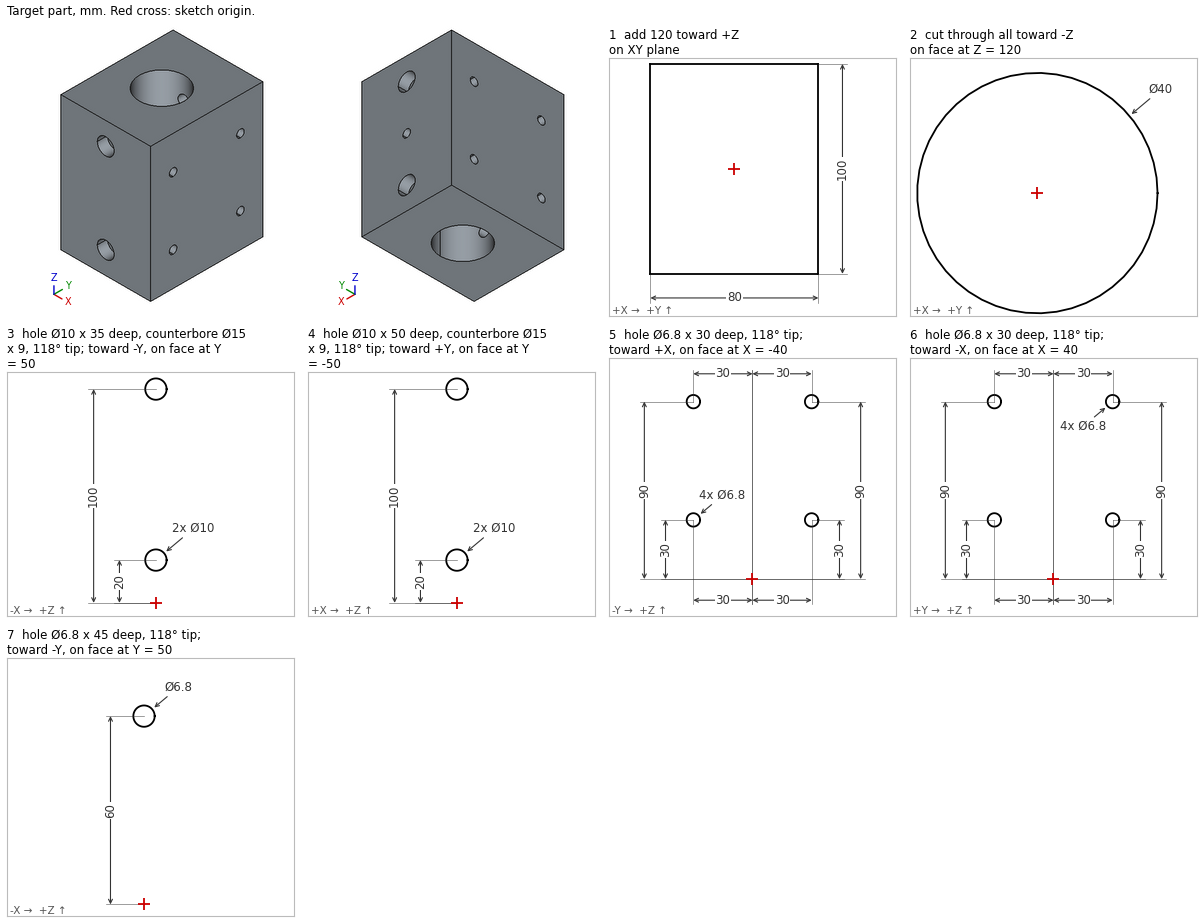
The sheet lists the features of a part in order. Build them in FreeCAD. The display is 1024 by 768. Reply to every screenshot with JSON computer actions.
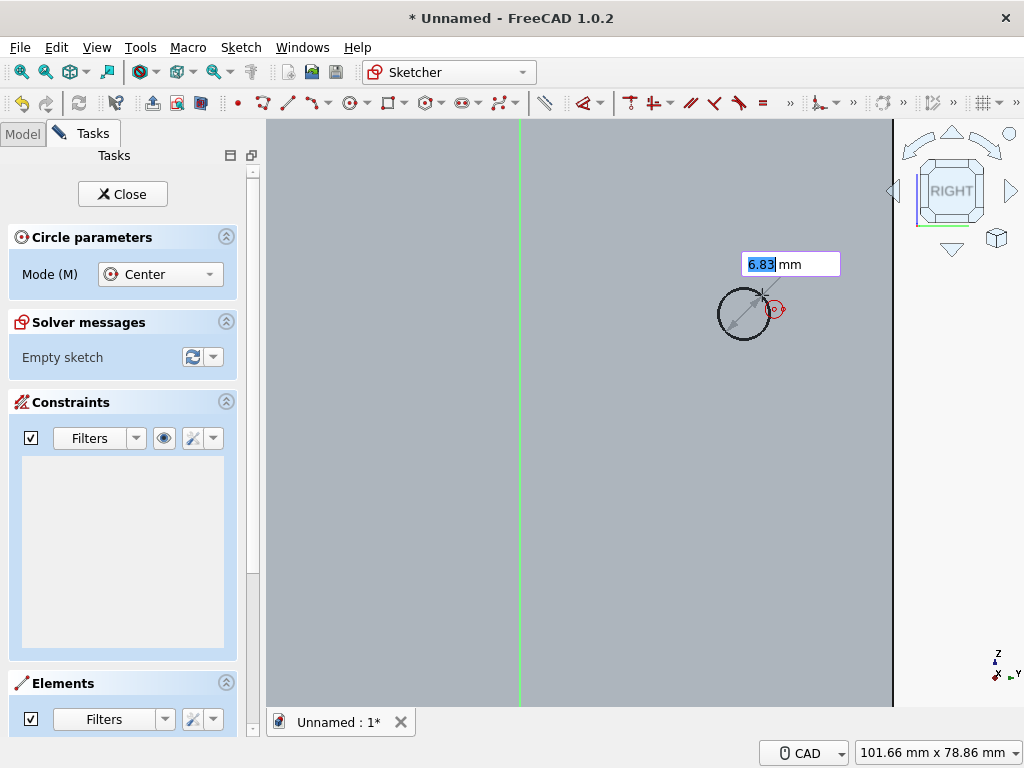
{"action": "type", "text": "6.8"}
{"action": "key", "text": "Return"}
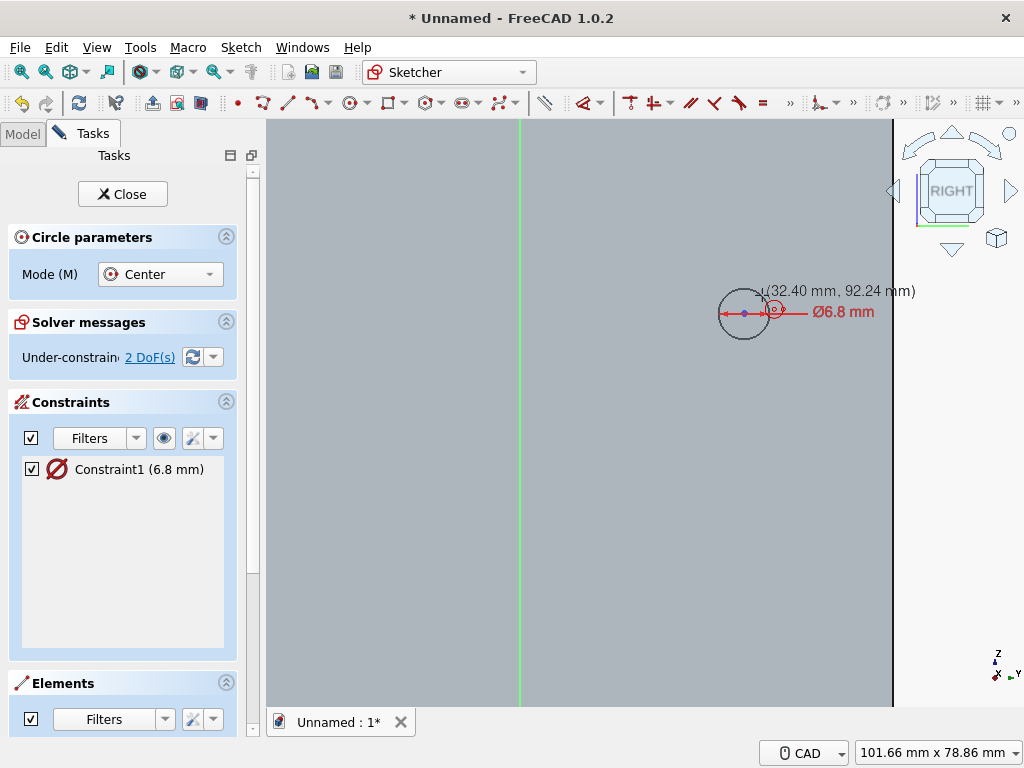
{"action": "scroll", "coordinate": [645, 147], "scroll_direction": "down", "scroll_amount": 3}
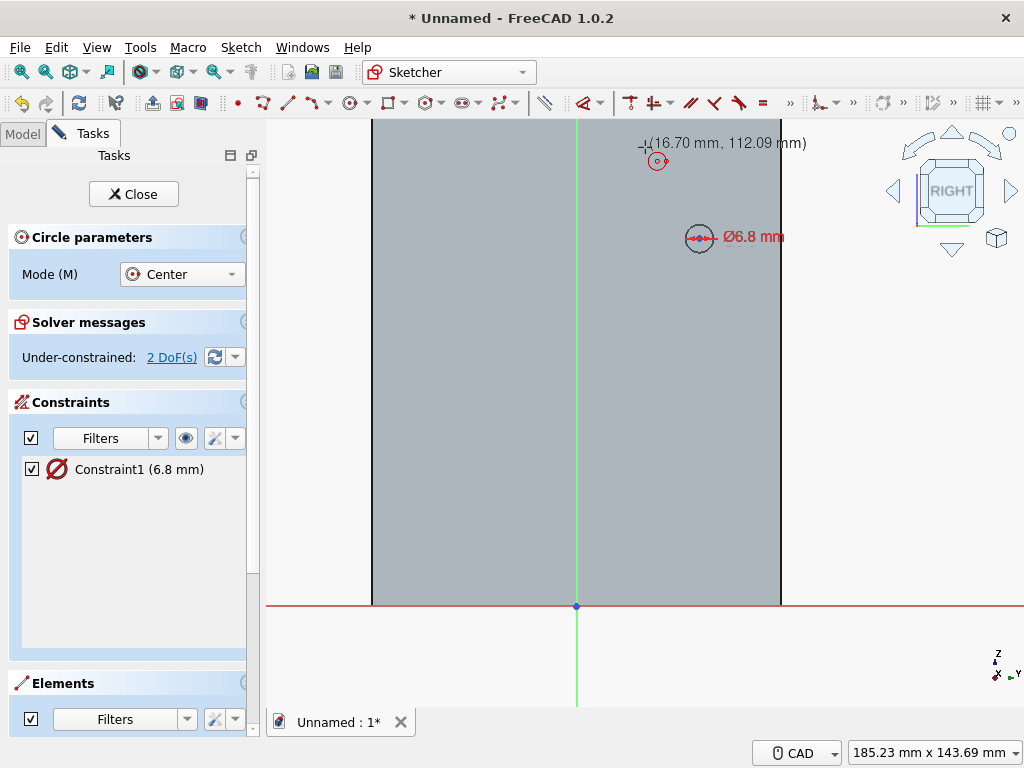
{"action": "scroll", "coordinate": [700, 483], "scroll_direction": "up", "scroll_amount": 3}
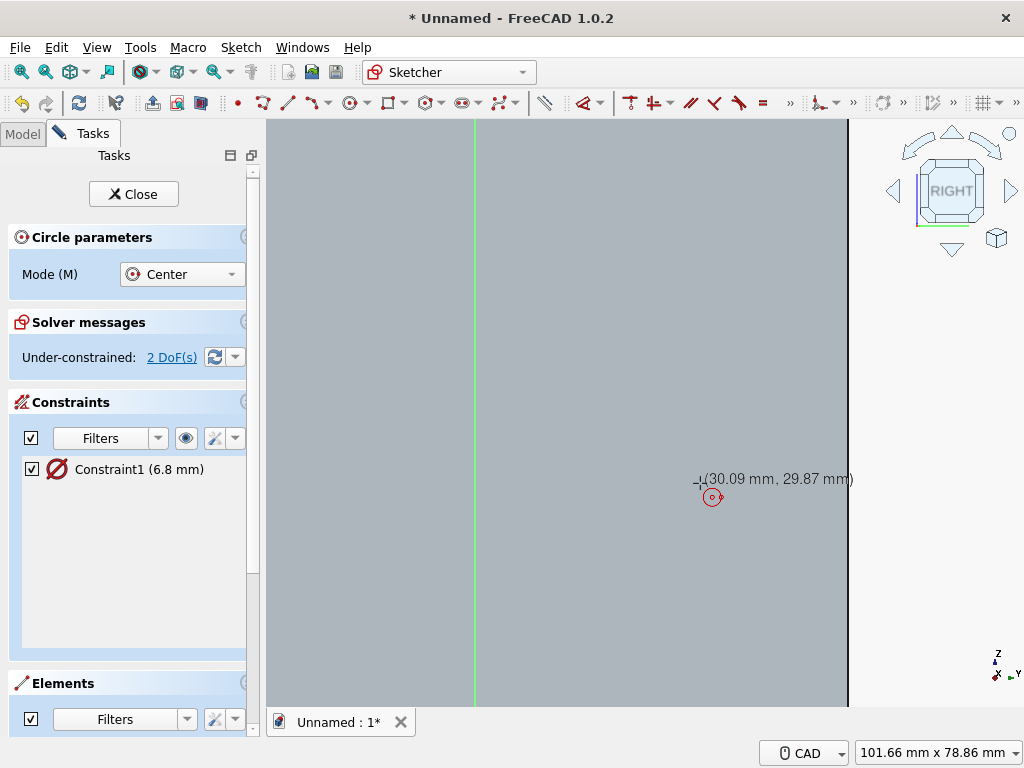
{"action": "left_click", "coordinate": [699, 483]}
{"action": "mouse_move", "coordinate": [717, 465]}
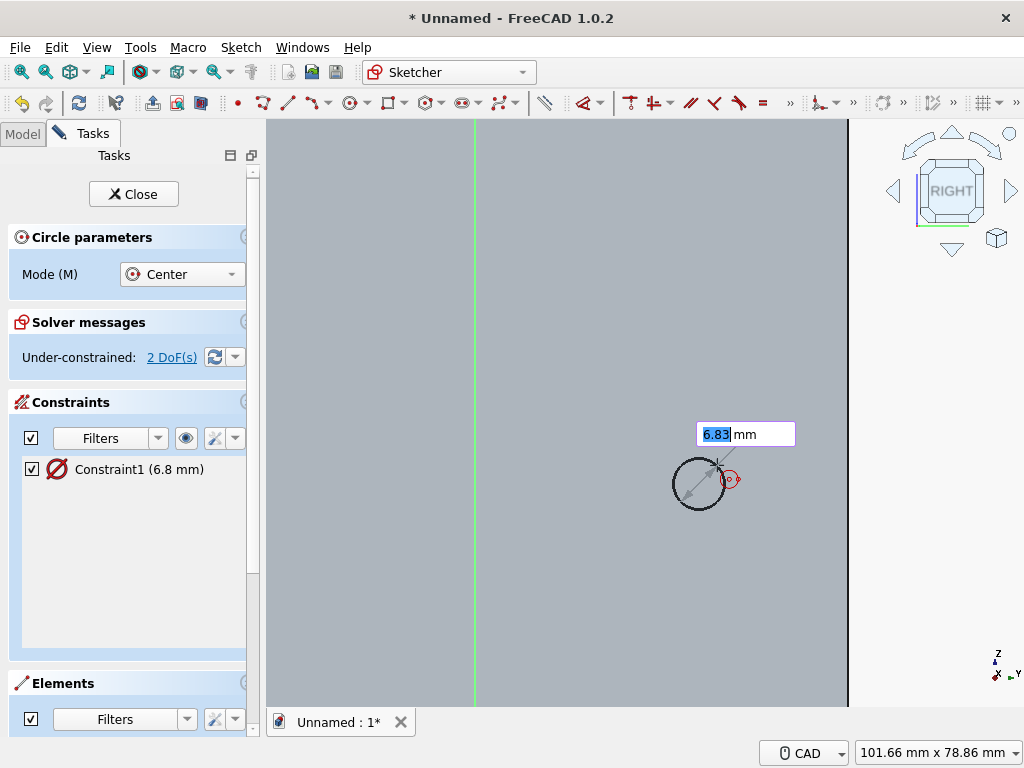
{"action": "type", "text": "6.8"}
{"action": "key", "text": "Return"}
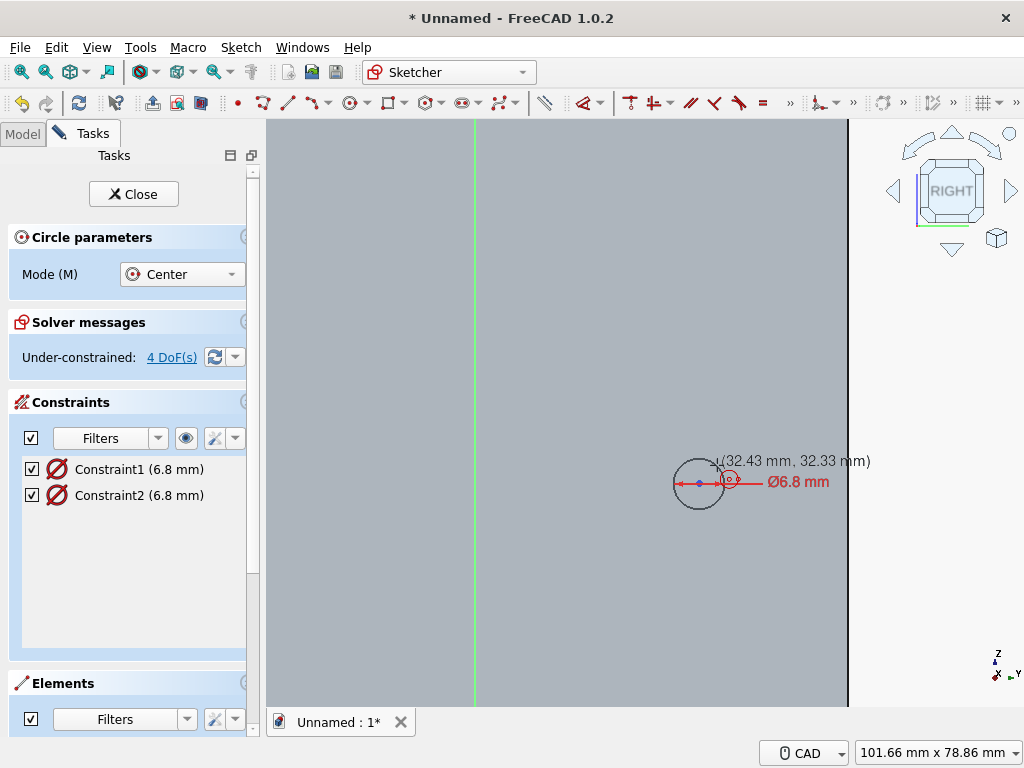
{"action": "scroll", "coordinate": [700, 479], "scroll_direction": "down", "scroll_amount": 3}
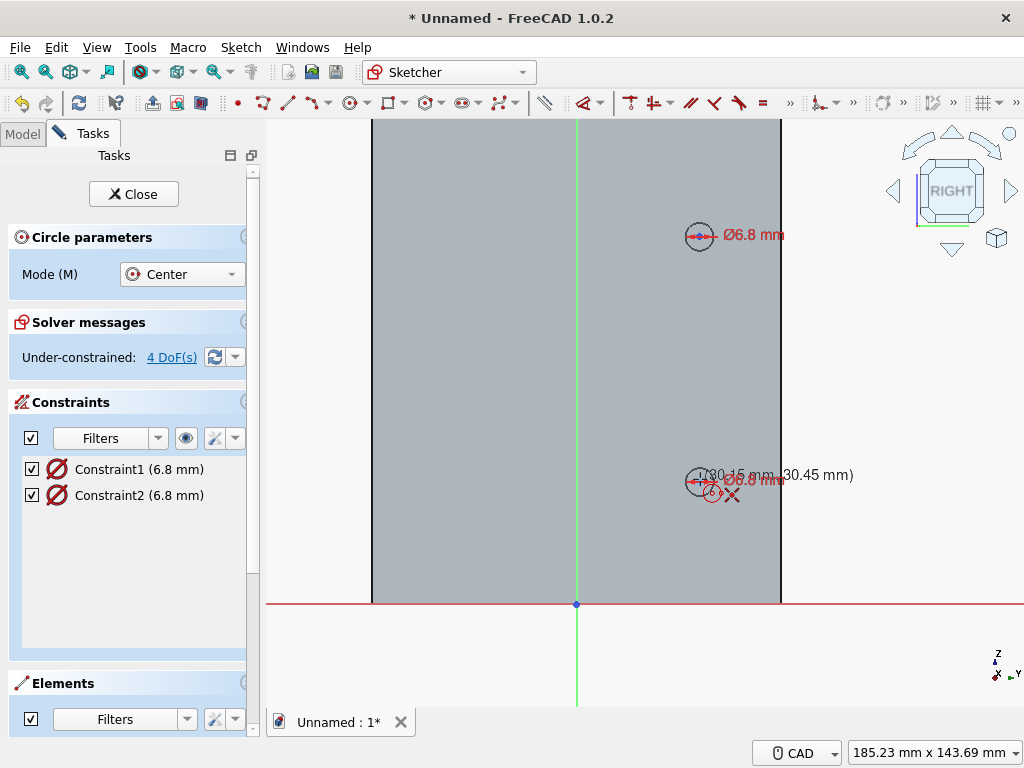
{"action": "scroll", "coordinate": [454, 482], "scroll_direction": "up", "scroll_amount": 3}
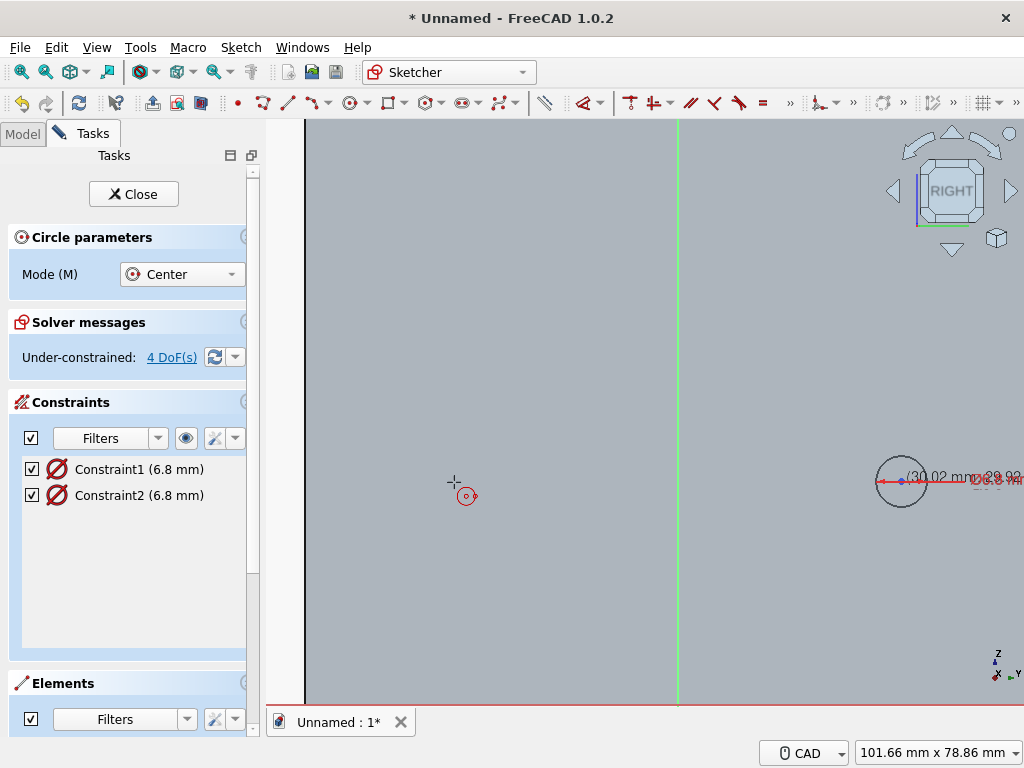
{"action": "left_click", "coordinate": [454, 481]}
{"action": "mouse_move", "coordinate": [472, 463]}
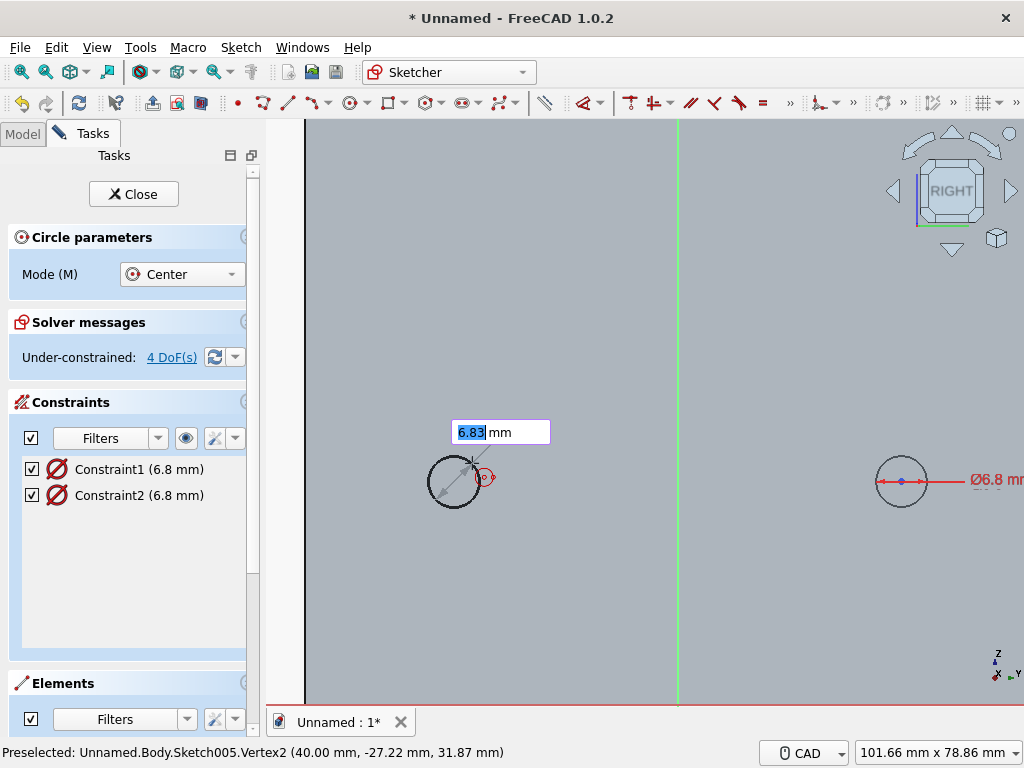
{"action": "type", "text": "6.8"}
{"action": "key", "text": "Return"}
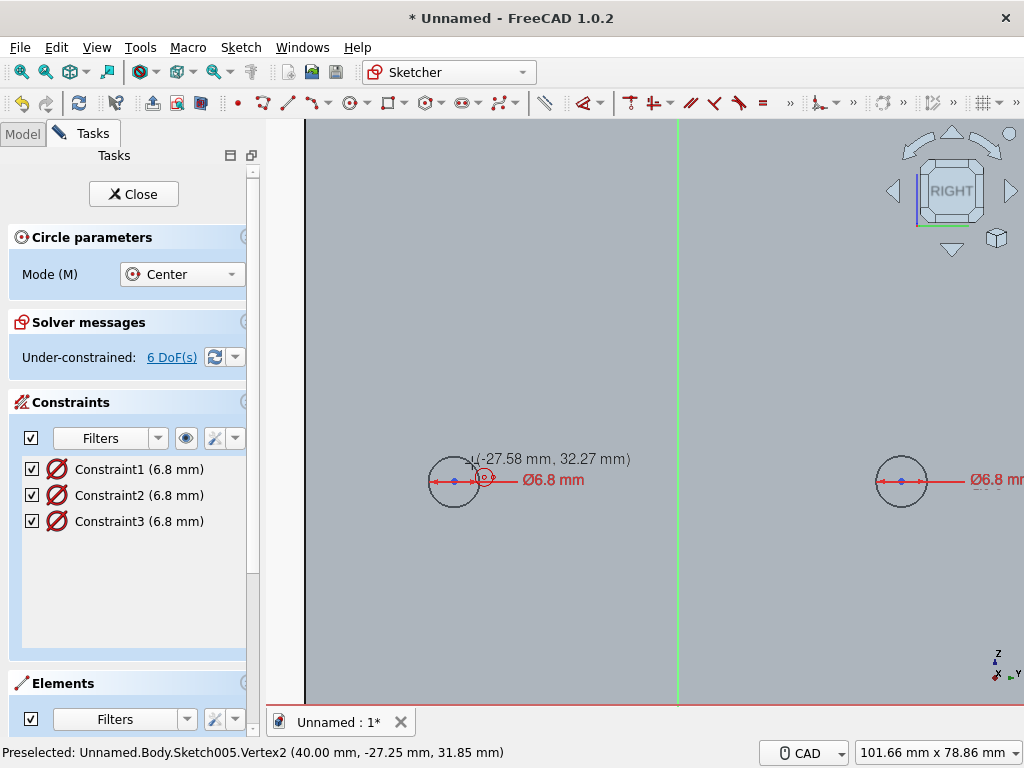
{"action": "scroll", "coordinate": [453, 482], "scroll_direction": "down", "scroll_amount": 3}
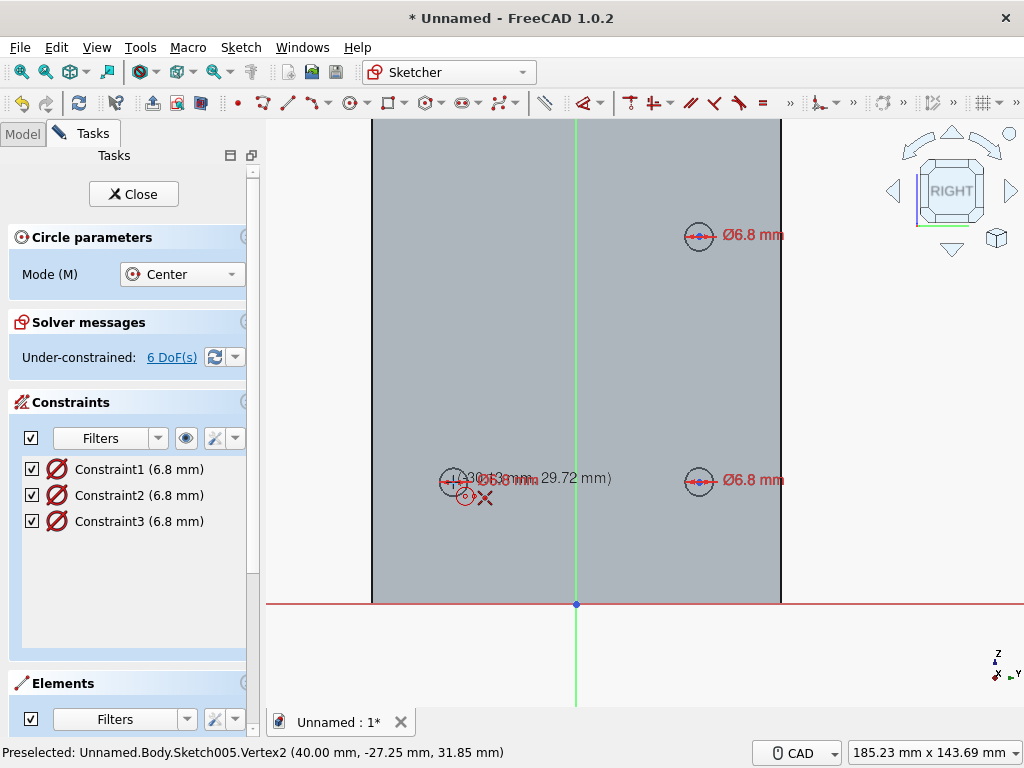
{"action": "scroll", "coordinate": [454, 236], "scroll_direction": "up", "scroll_amount": 3}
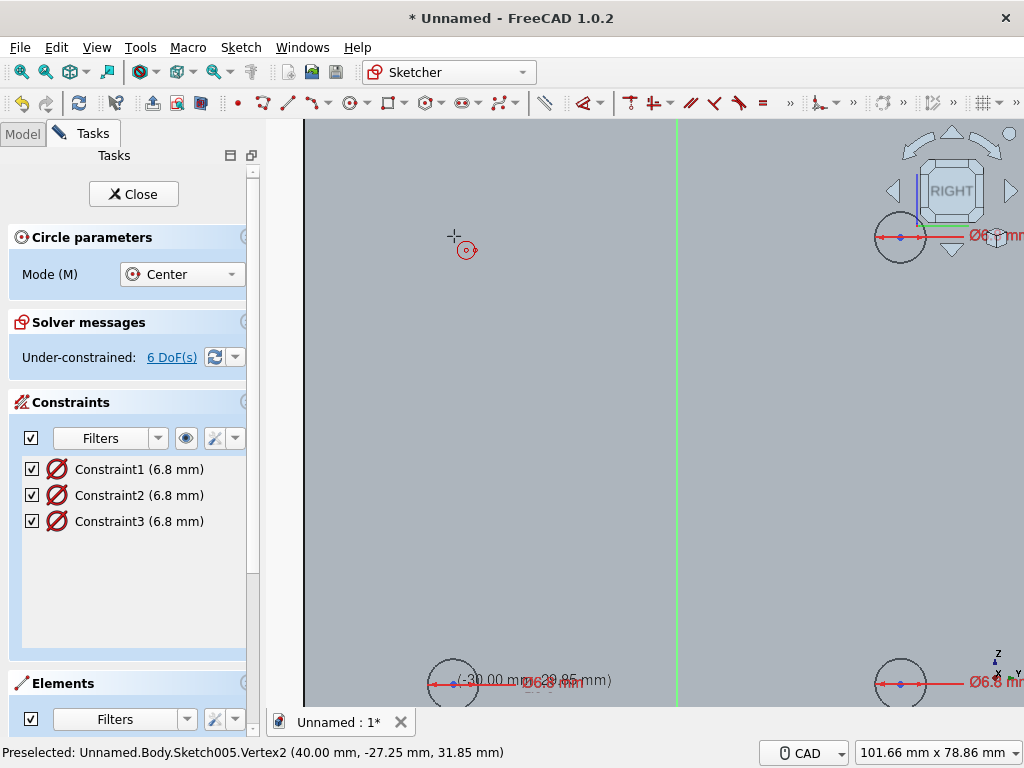
{"action": "left_click", "coordinate": [453, 236]}
{"action": "mouse_move", "coordinate": [471, 218]}